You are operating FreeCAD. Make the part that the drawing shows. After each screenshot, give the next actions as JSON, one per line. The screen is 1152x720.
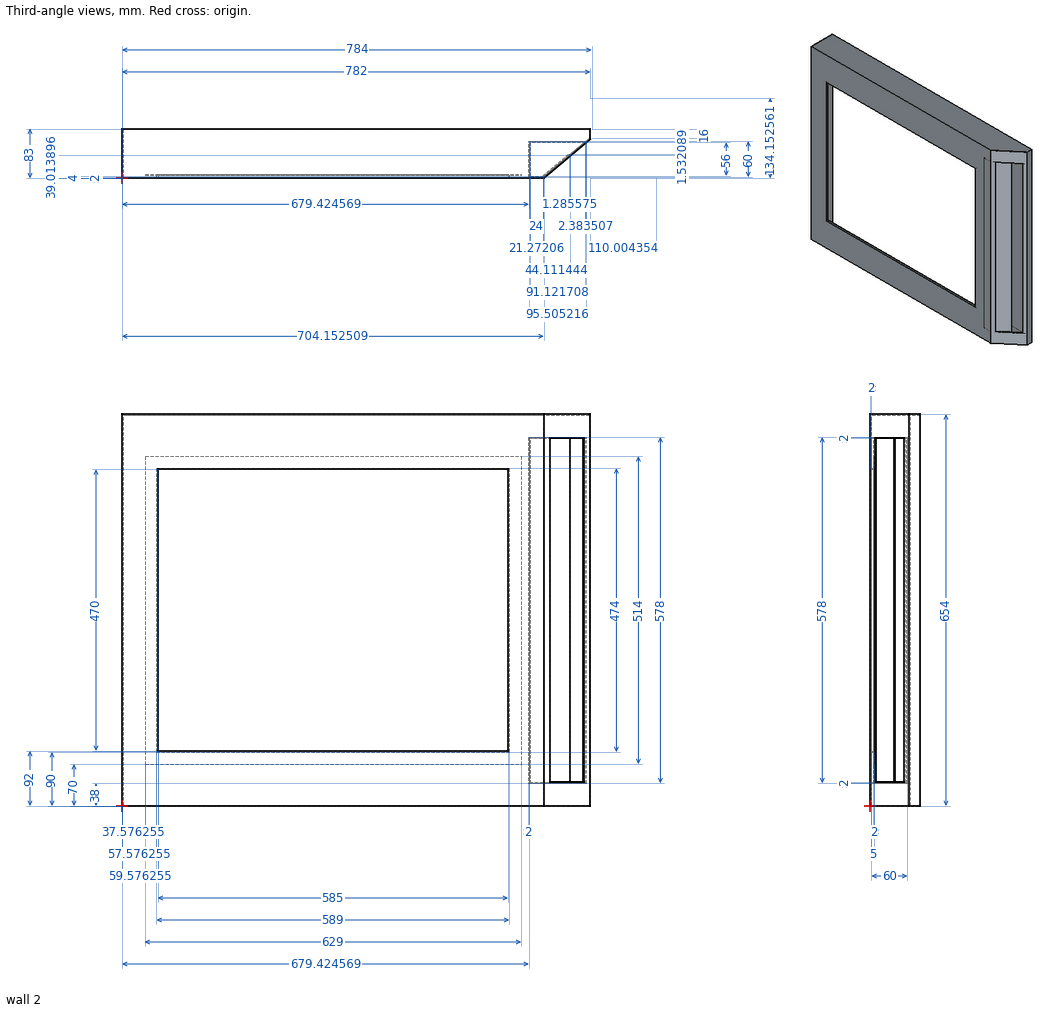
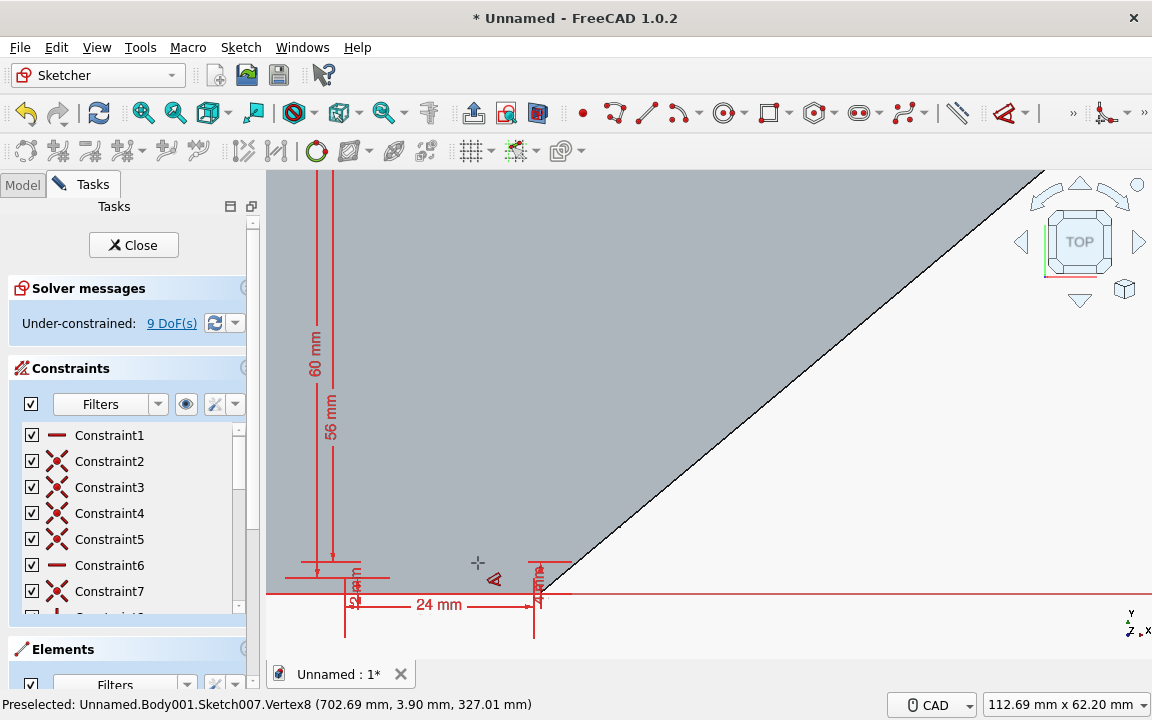
{"action": "left_click", "coordinate": [478, 562]}
{"action": "left_click", "coordinate": [444, 528]}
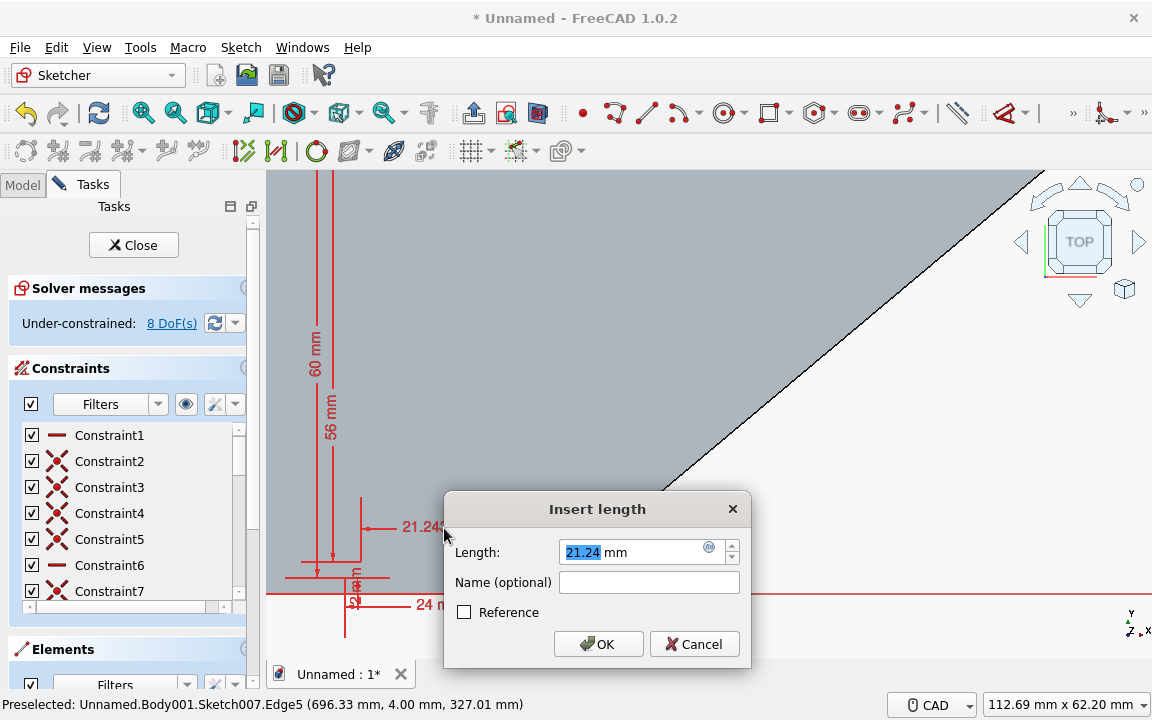
{"action": "type", "text": "21.27206"}
{"action": "key", "text": "Return"}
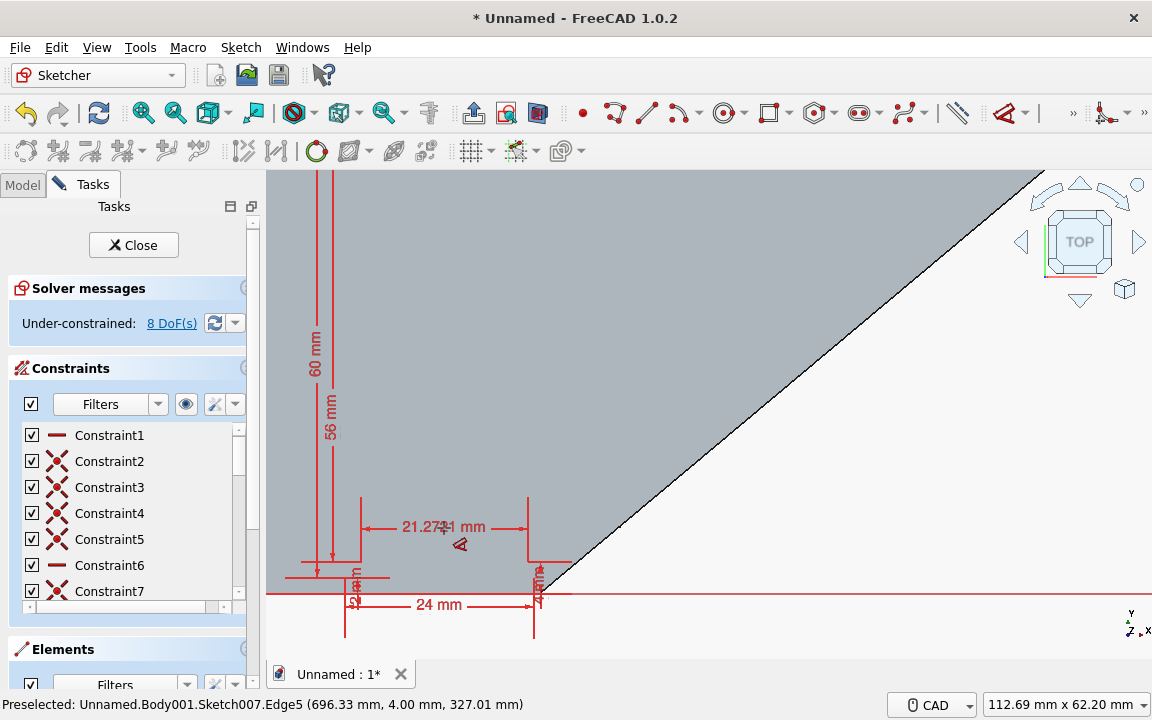
{"action": "scroll", "coordinate": [478, 562], "scroll_direction": "down", "scroll_amount": 2}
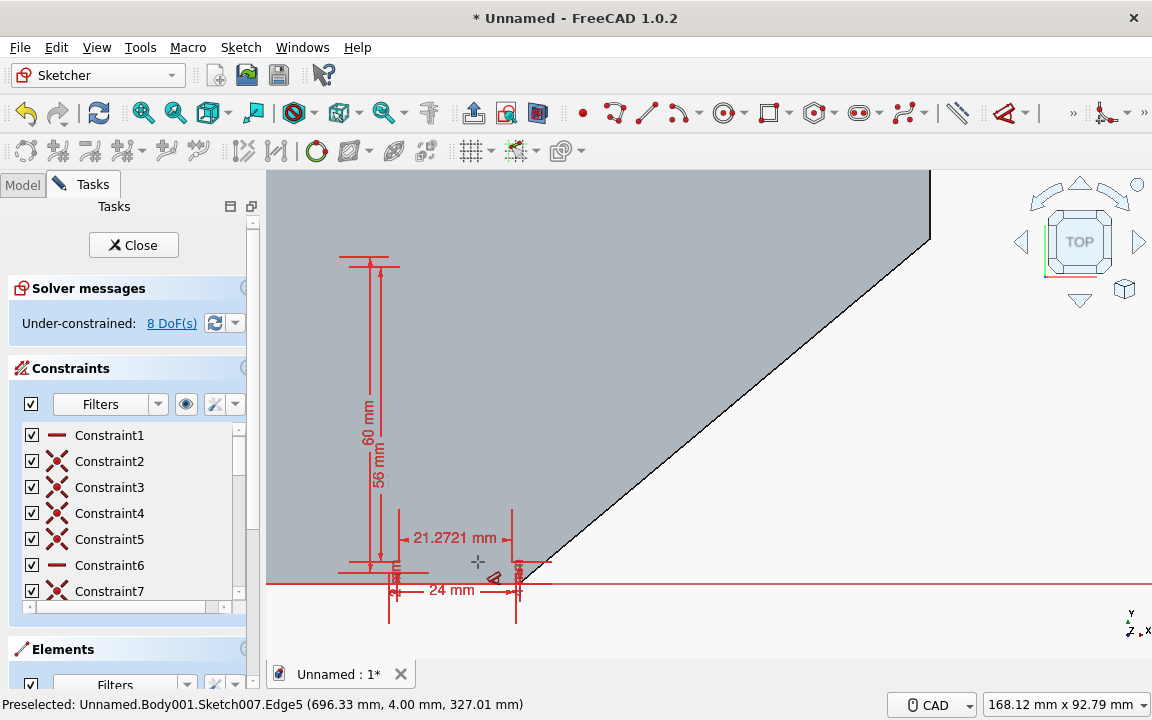
{"action": "scroll", "coordinate": [544, 267], "scroll_direction": "up", "scroll_amount": 2}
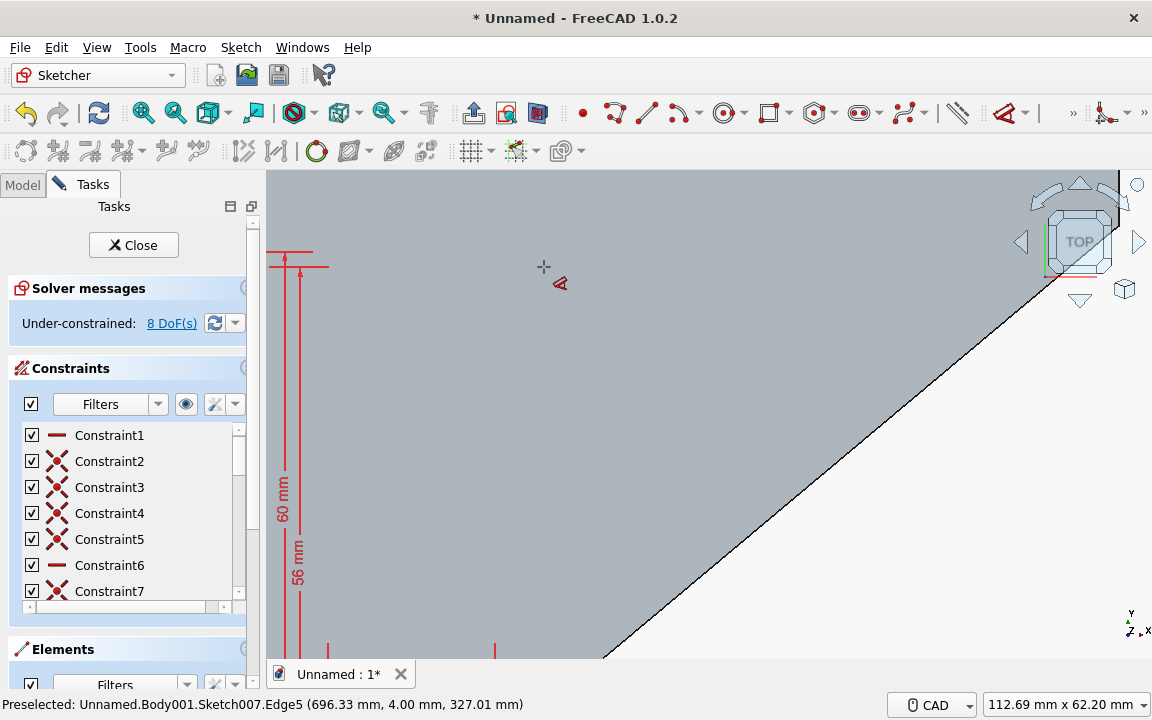
{"action": "left_click", "coordinate": [543, 267]}
{"action": "left_click", "coordinate": [658, 233]}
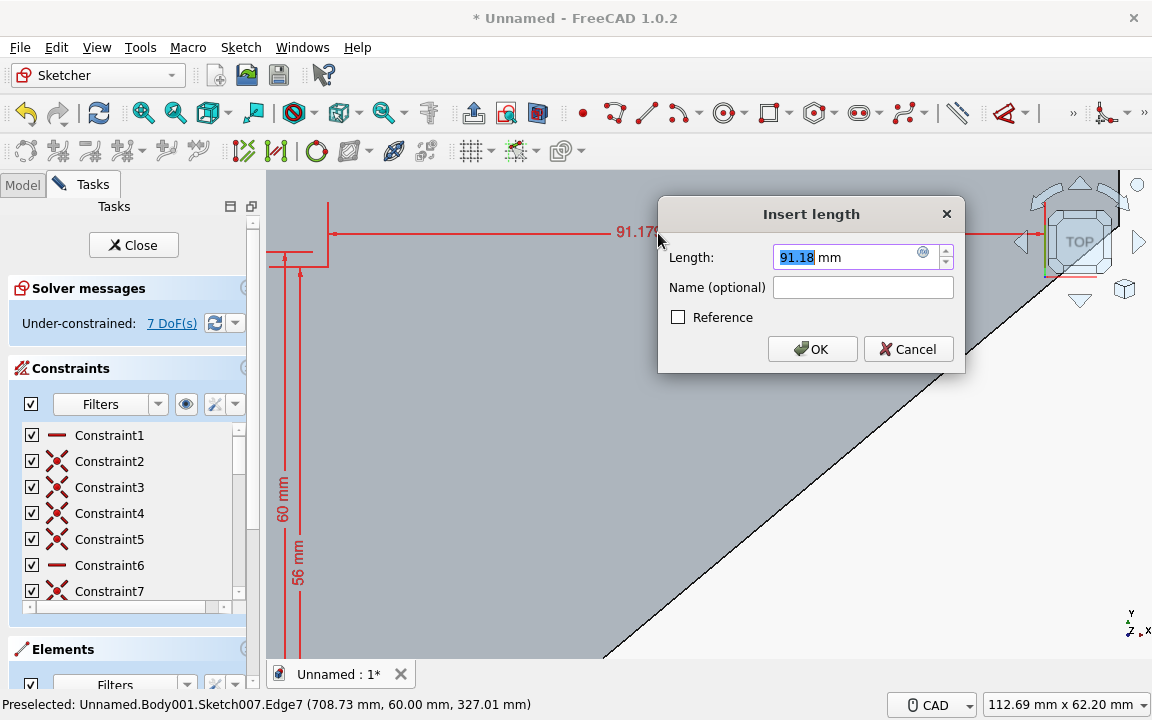
{"action": "type", "text": "91.121708"}
{"action": "key", "text": "Return"}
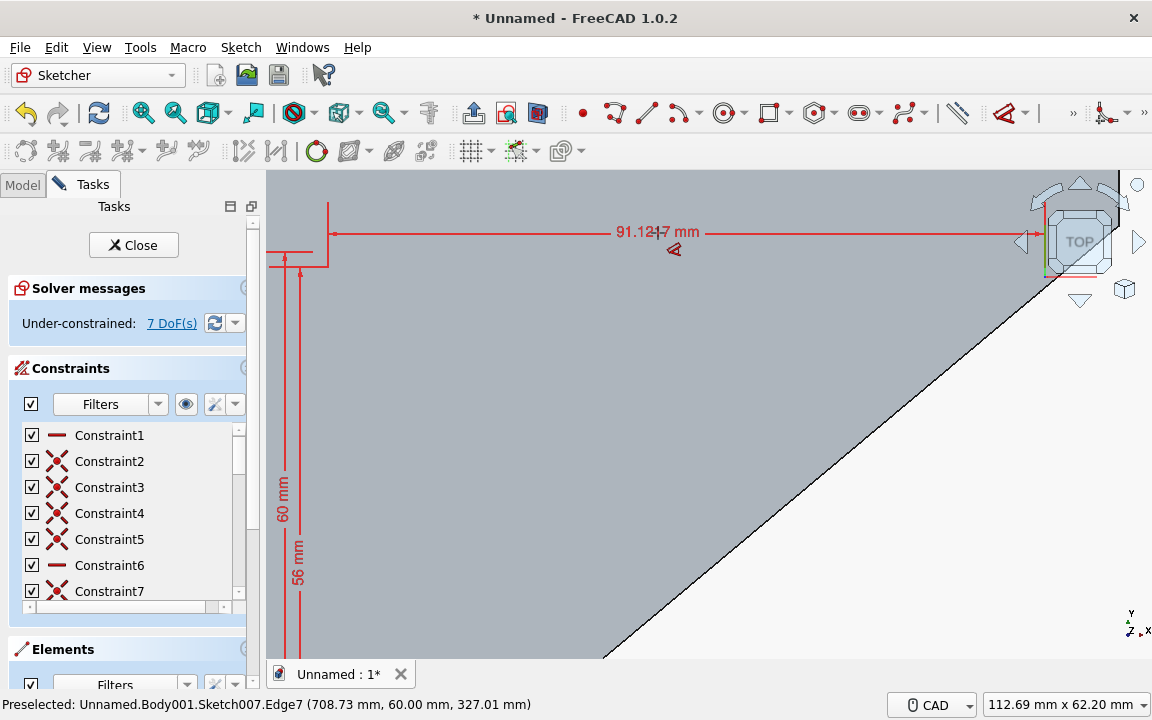
{"action": "left_click", "coordinate": [838, 252]}
{"action": "left_click", "coordinate": [495, 218]}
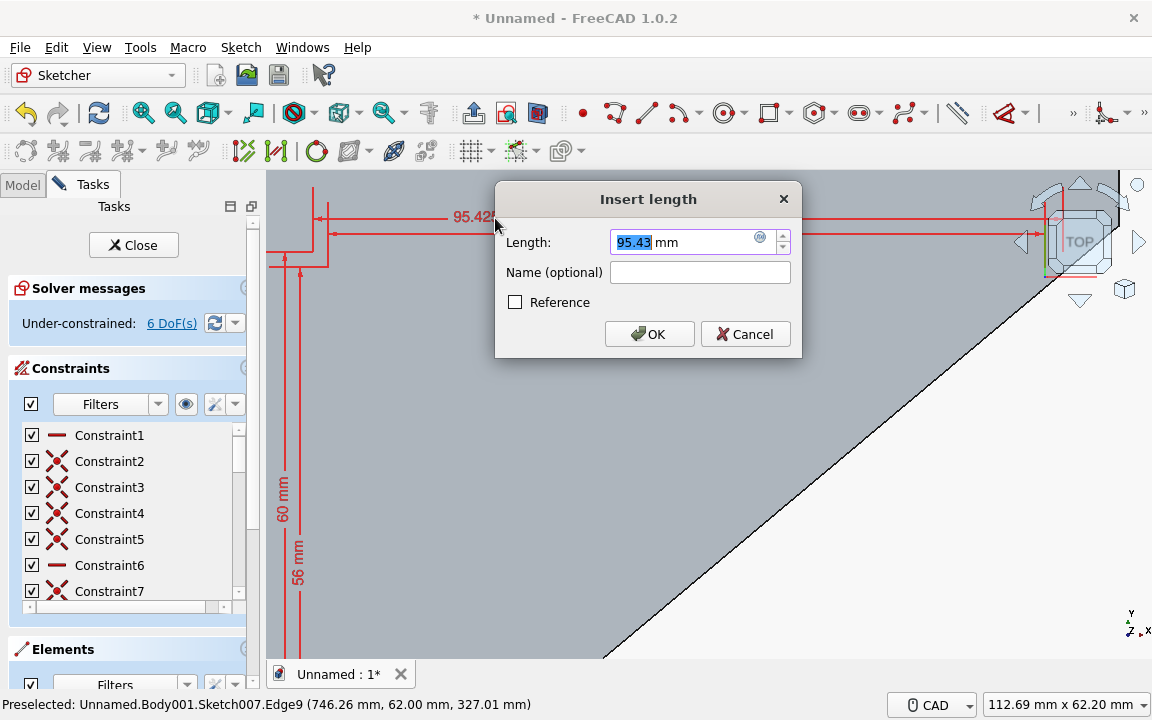
{"action": "type", "text": "95.505216"}
{"action": "key", "text": "Return"}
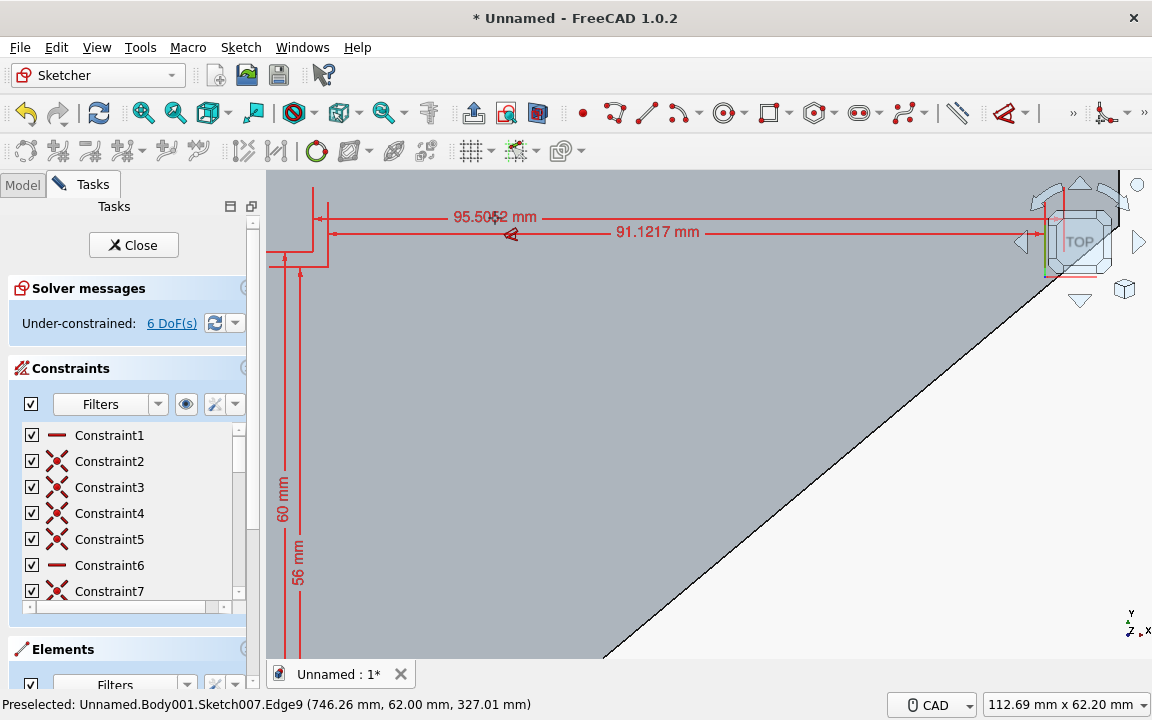
{"action": "scroll", "coordinate": [843, 428], "scroll_direction": "up", "scroll_amount": 7}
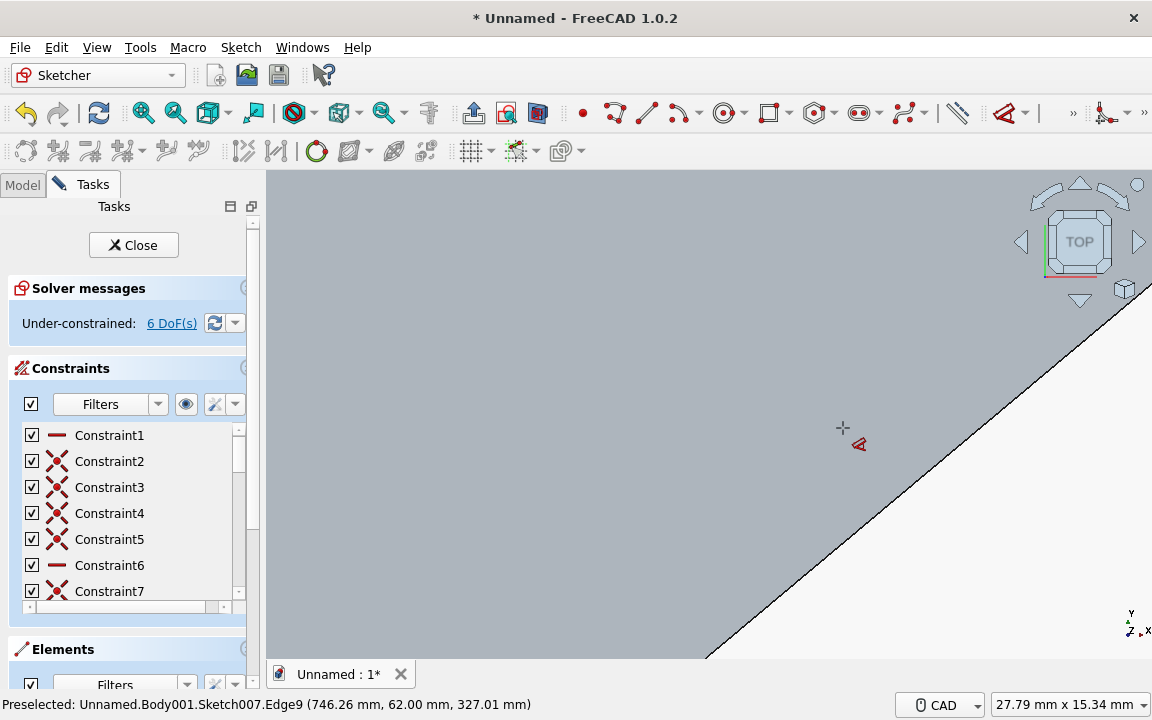
{"action": "left_click", "coordinate": [842, 425]}
{"action": "left_click", "coordinate": [842, 364]}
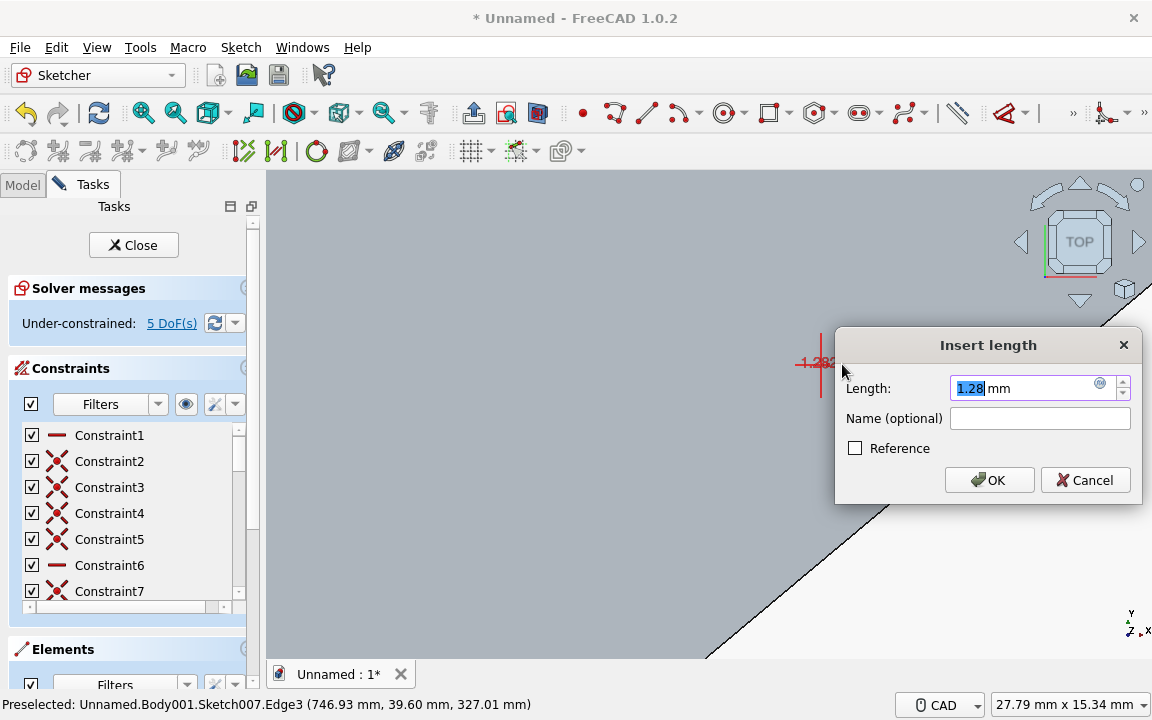
{"action": "type", "text": "1.285575"}
{"action": "key", "text": "Return"}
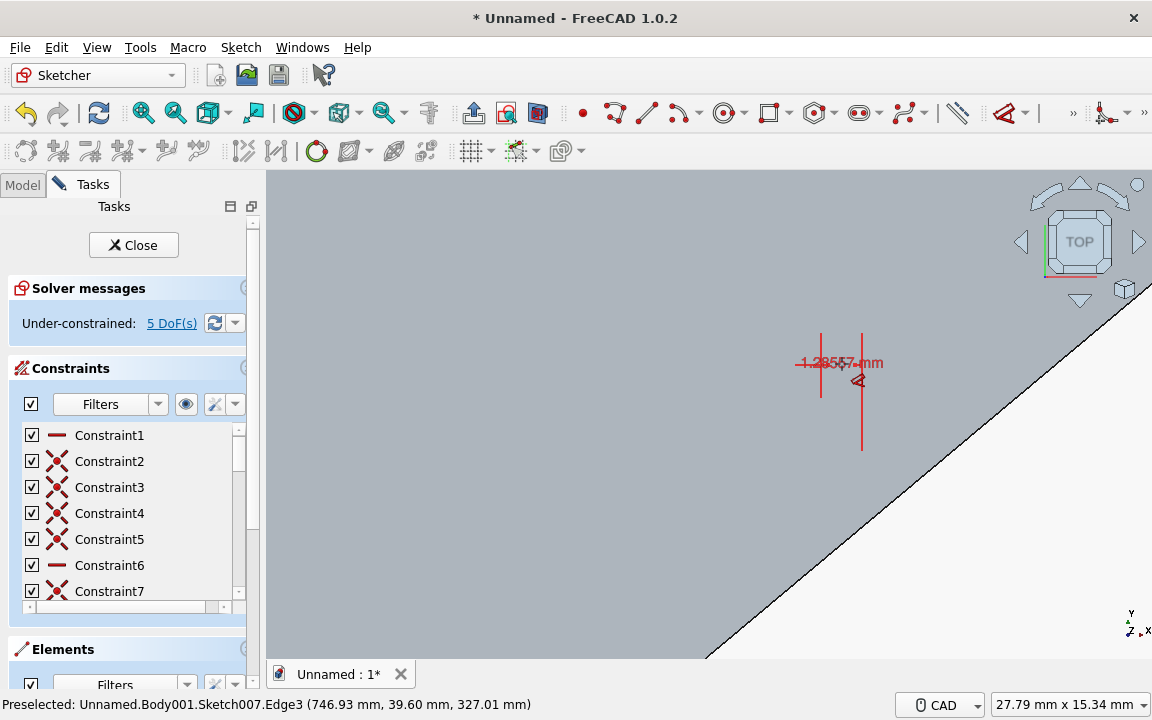
{"action": "left_click", "coordinate": [850, 435]}
{"action": "left_click", "coordinate": [896, 425]}